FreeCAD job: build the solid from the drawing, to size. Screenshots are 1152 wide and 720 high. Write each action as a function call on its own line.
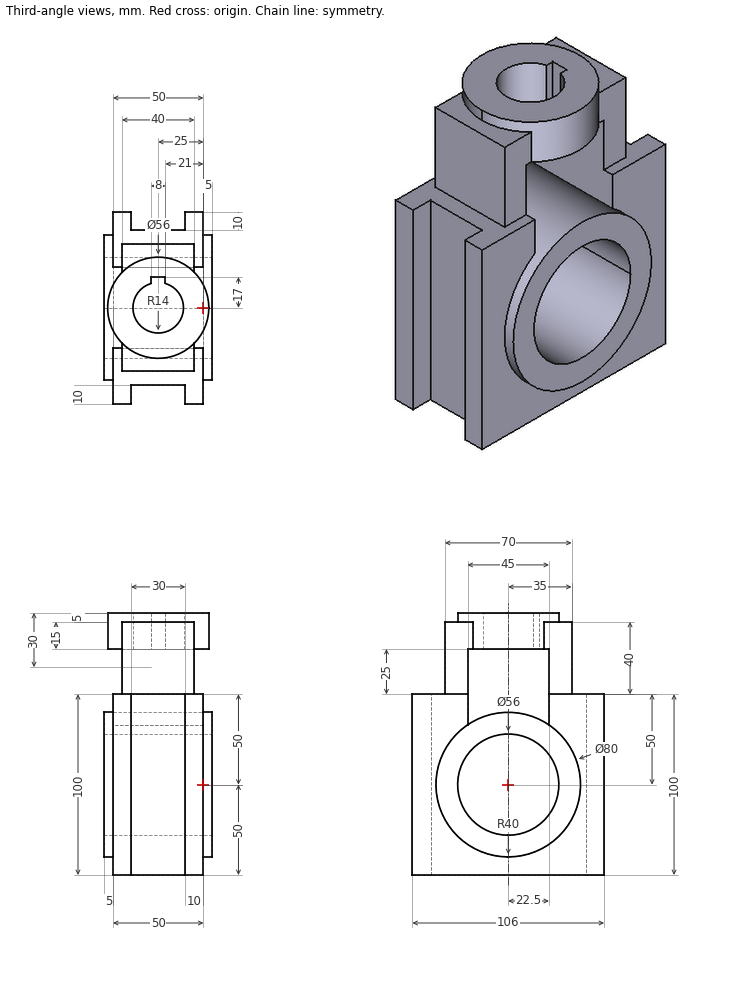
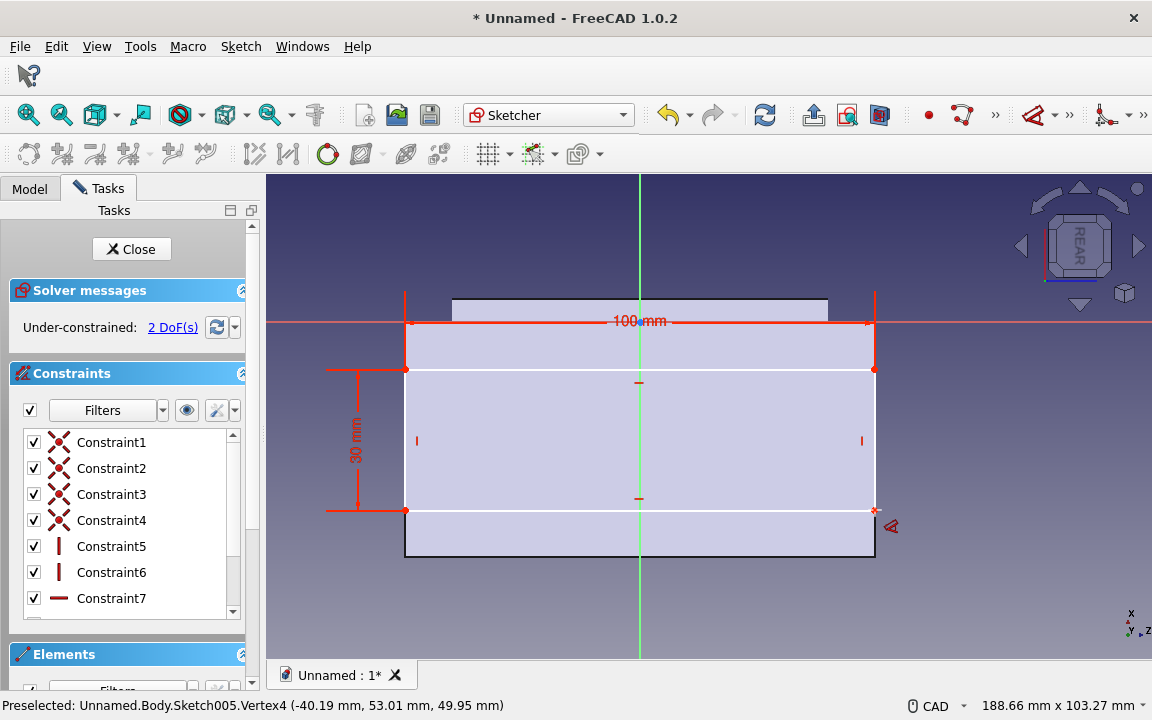
click(405, 370)
click(523, 288)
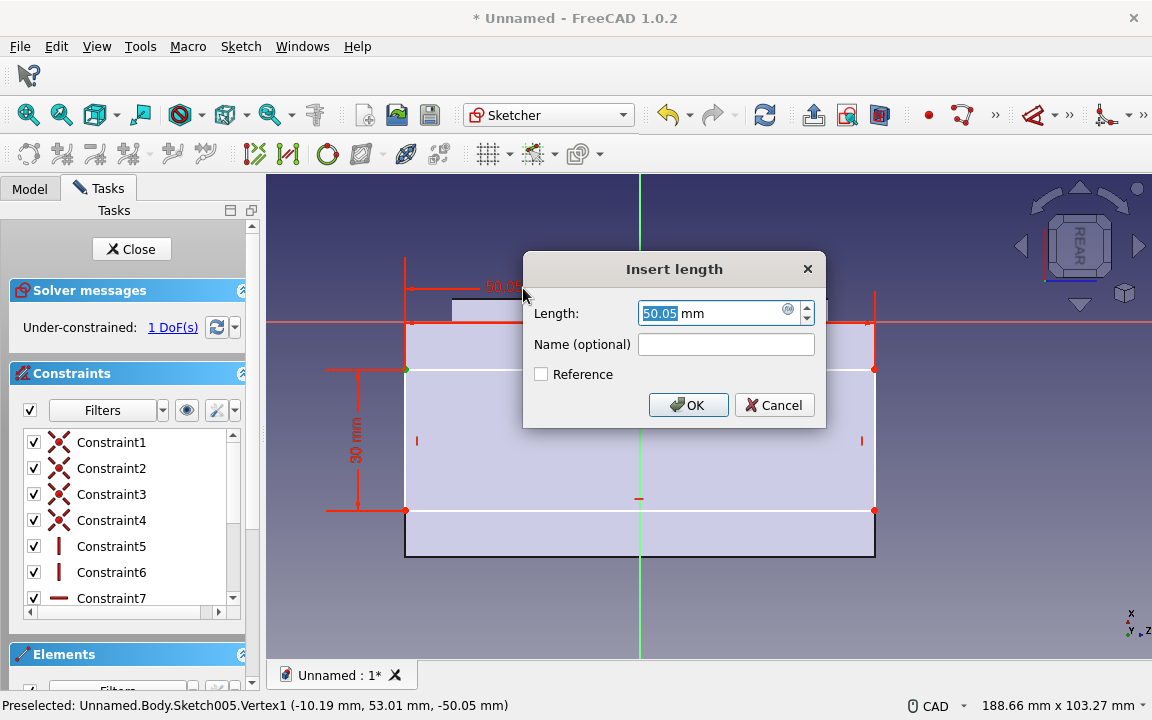
text(50)
key(Return)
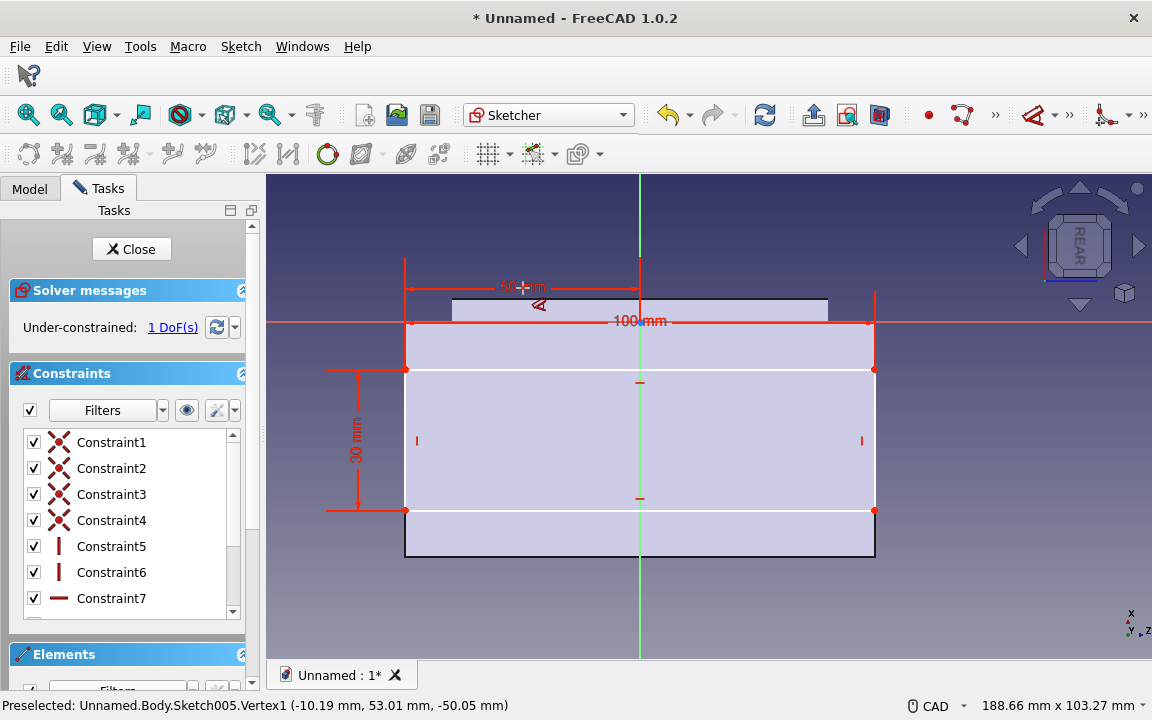
click(405, 370)
click(371, 346)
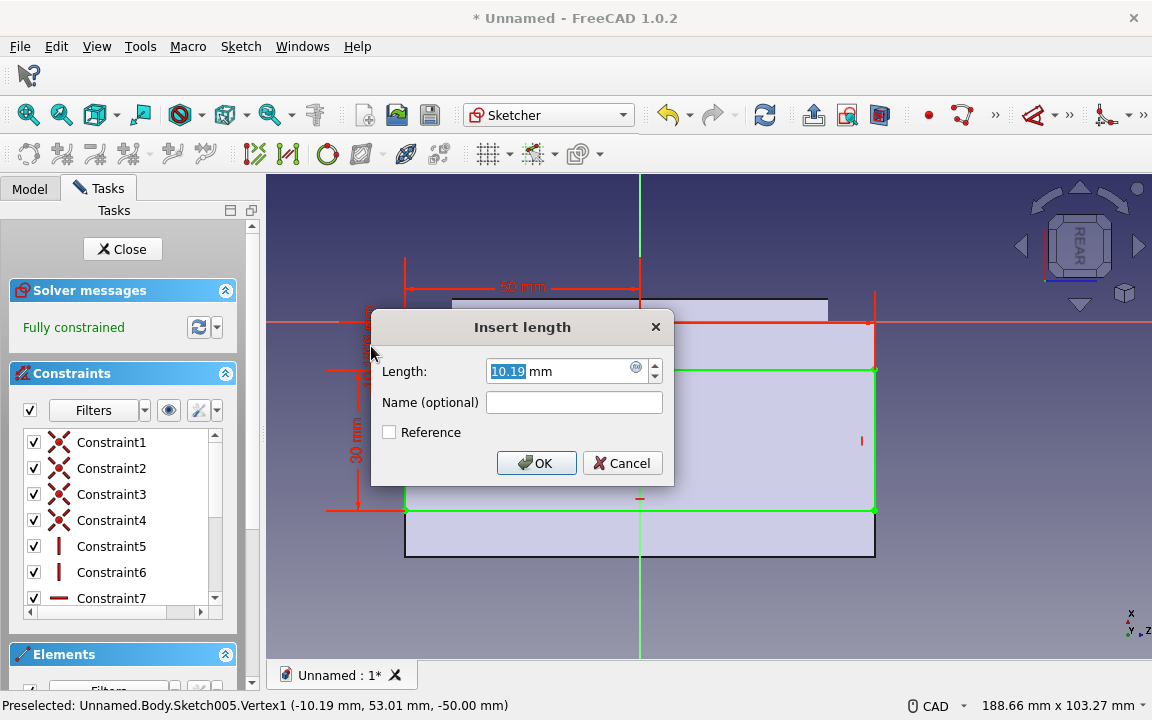
text(10)
key(Return)
key(Escape)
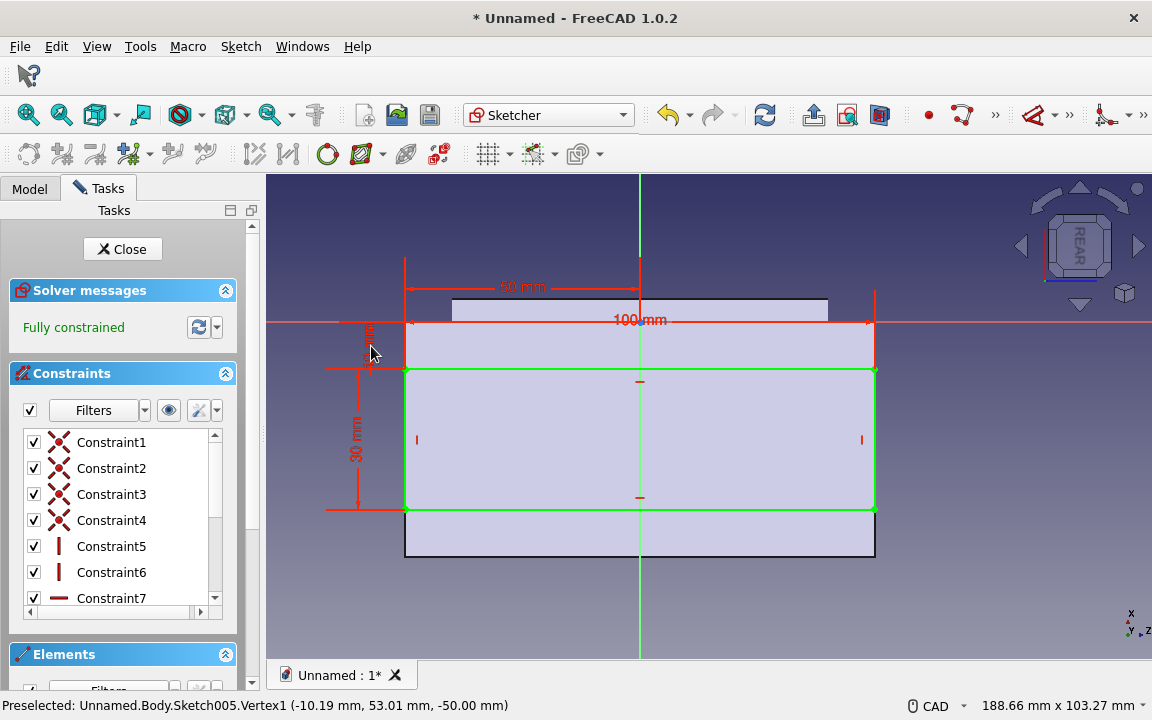
click(123, 249)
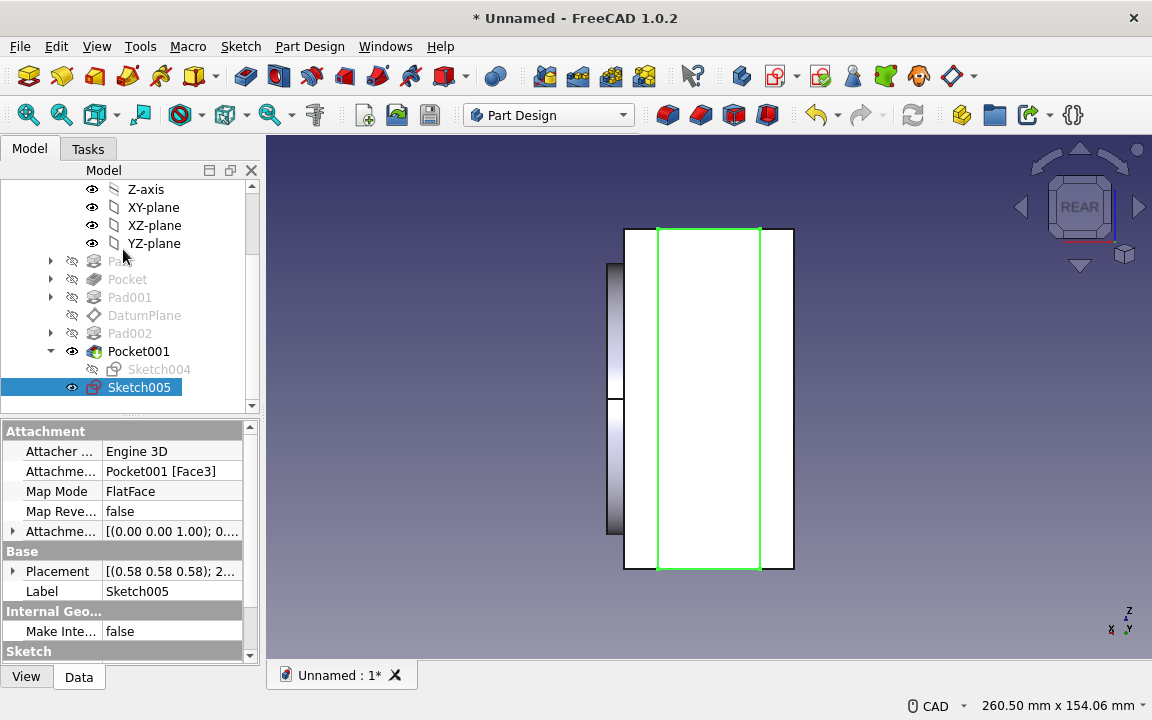
click(246, 76)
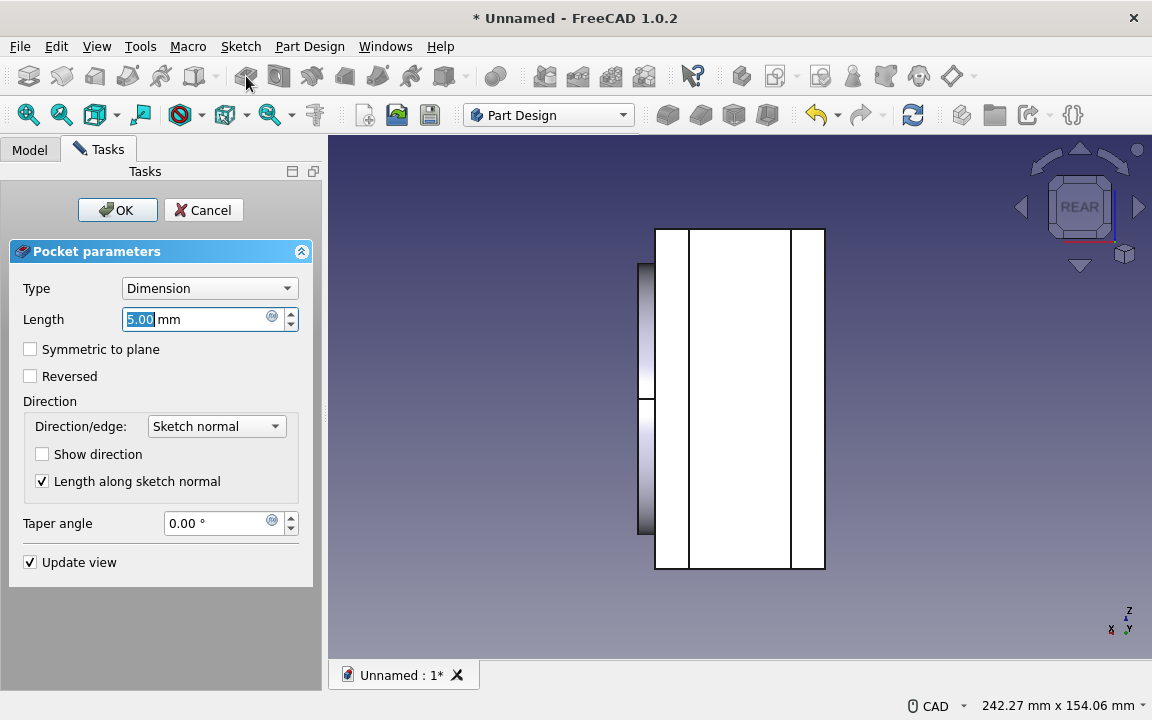
text(10)
key(Tab)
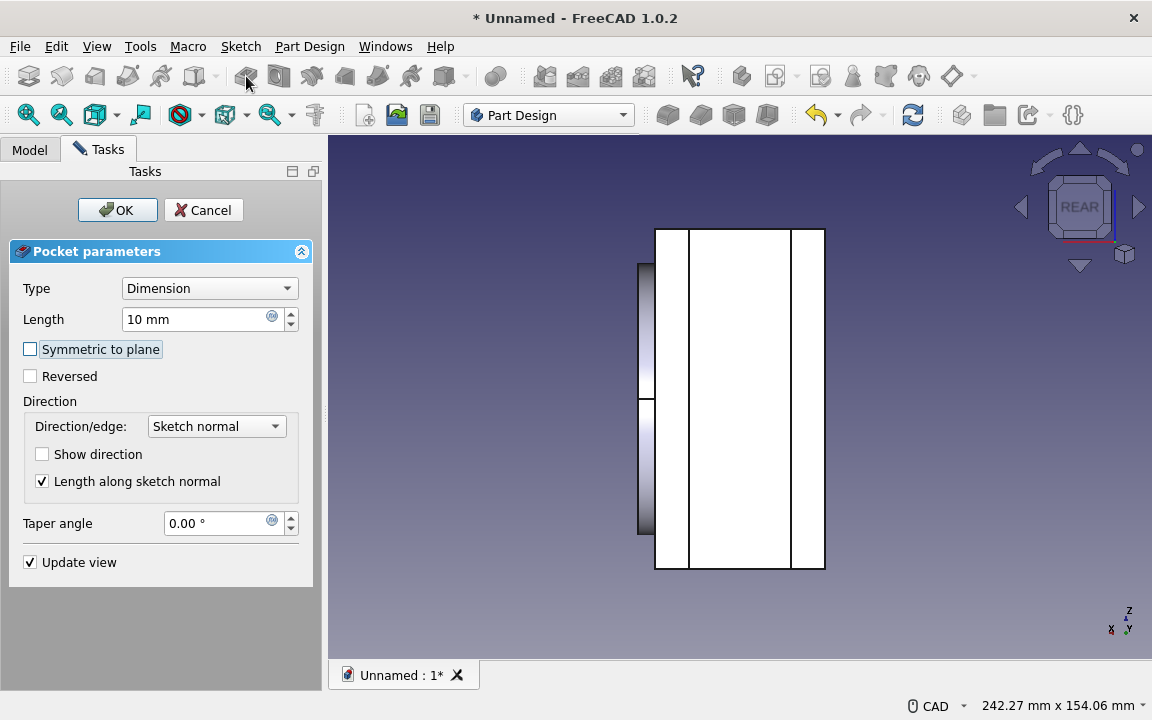
click(118, 210)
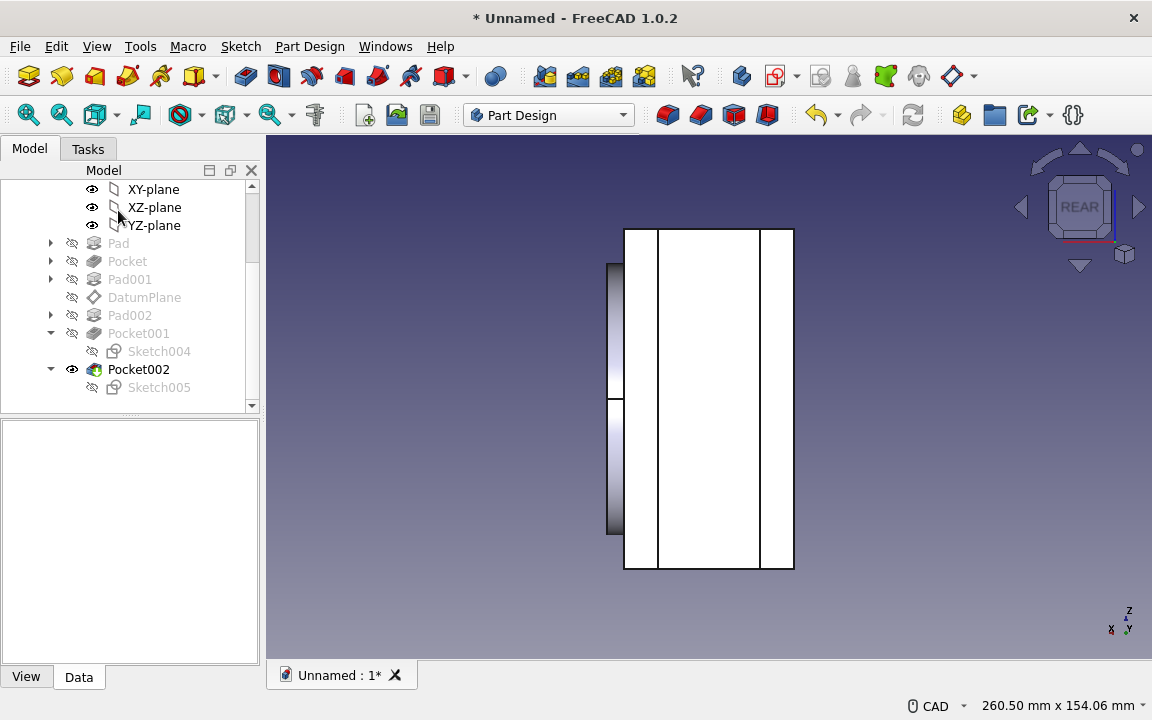
scroll(161, 293, down, 3)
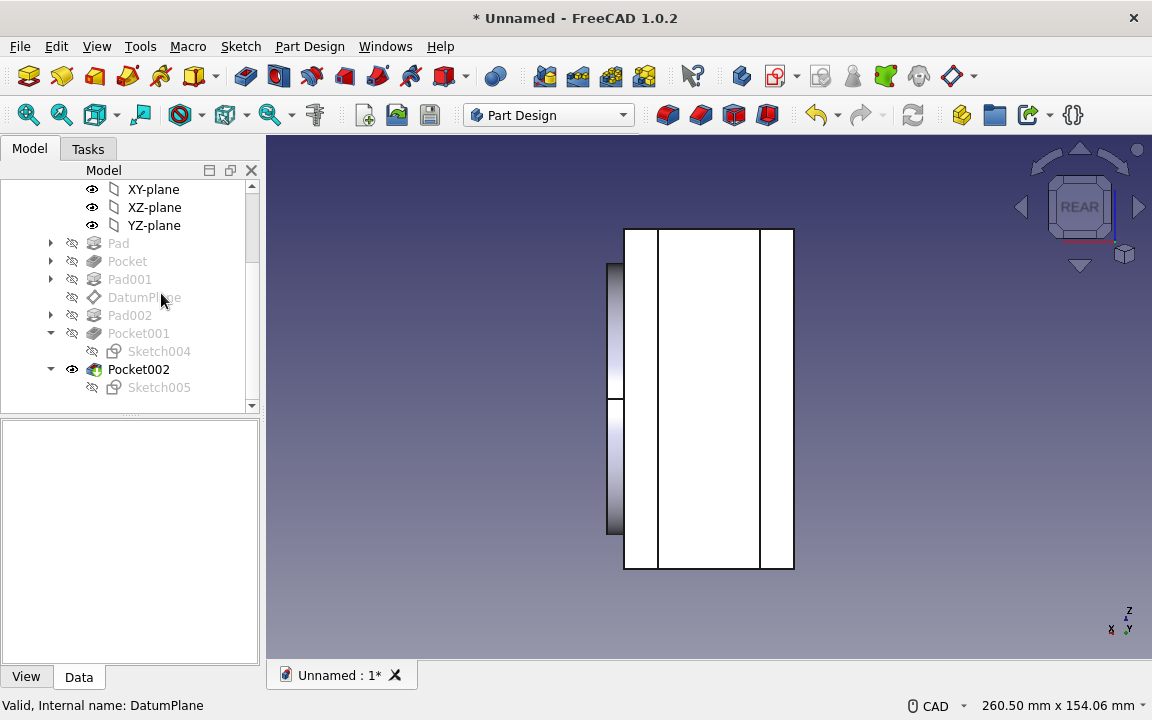
scroll(161, 293, up, 15)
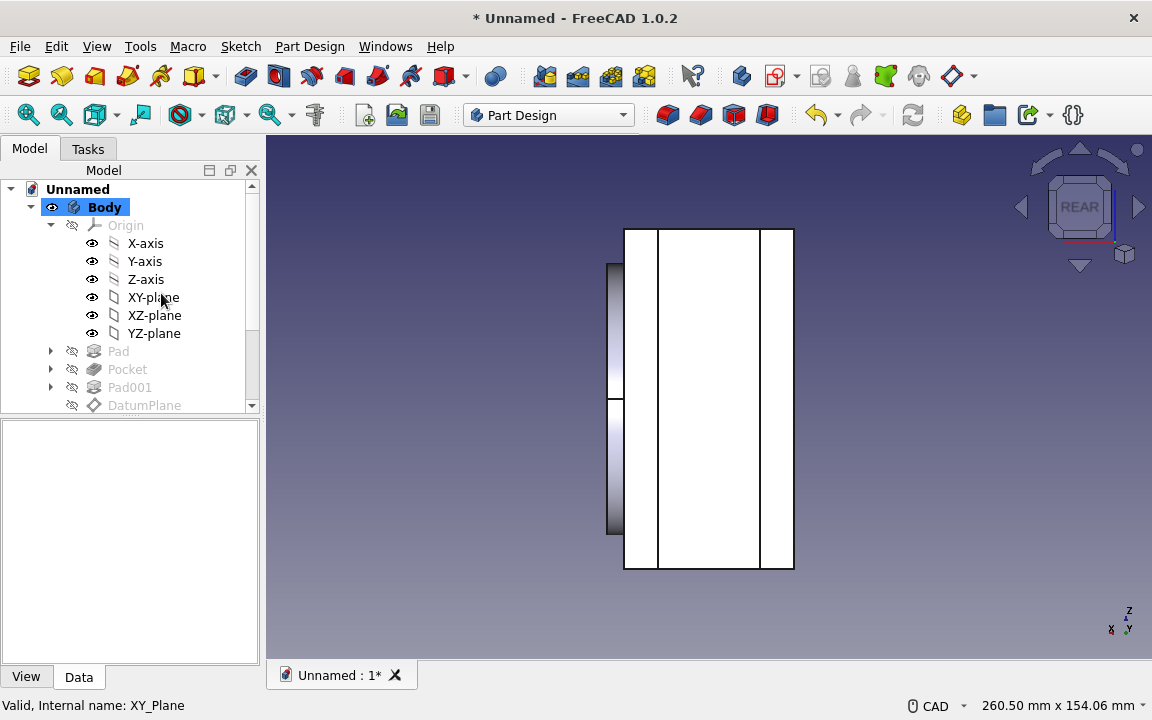
click(137, 333)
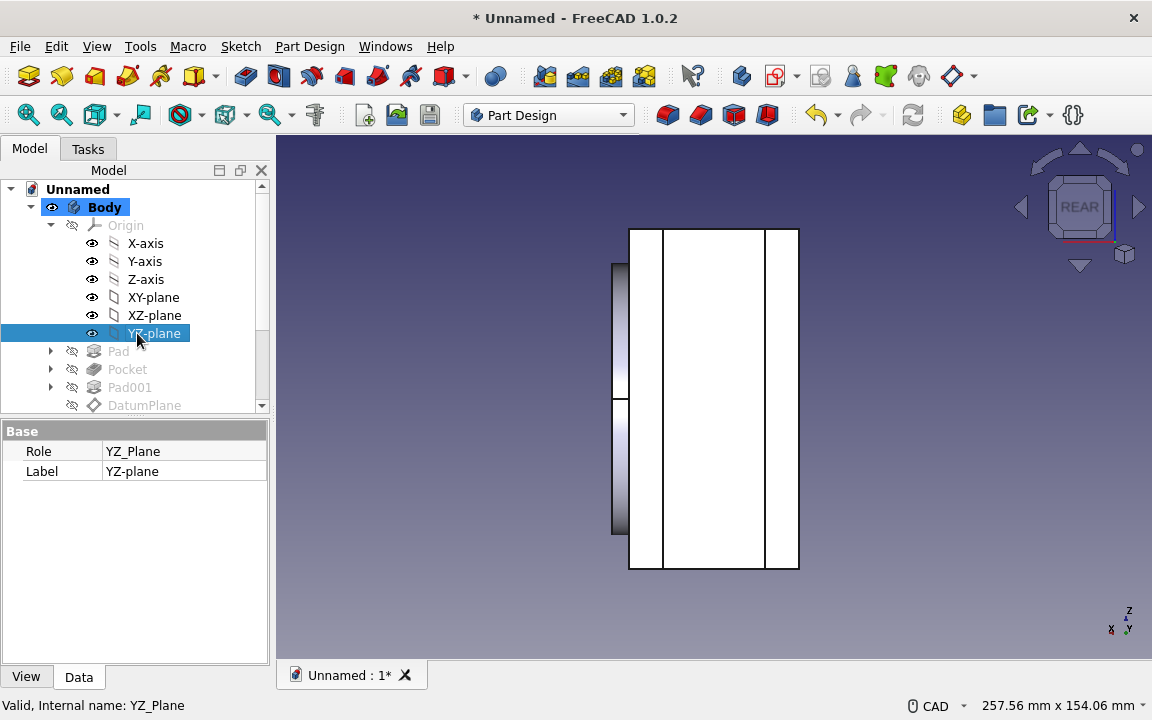
click(952, 76)